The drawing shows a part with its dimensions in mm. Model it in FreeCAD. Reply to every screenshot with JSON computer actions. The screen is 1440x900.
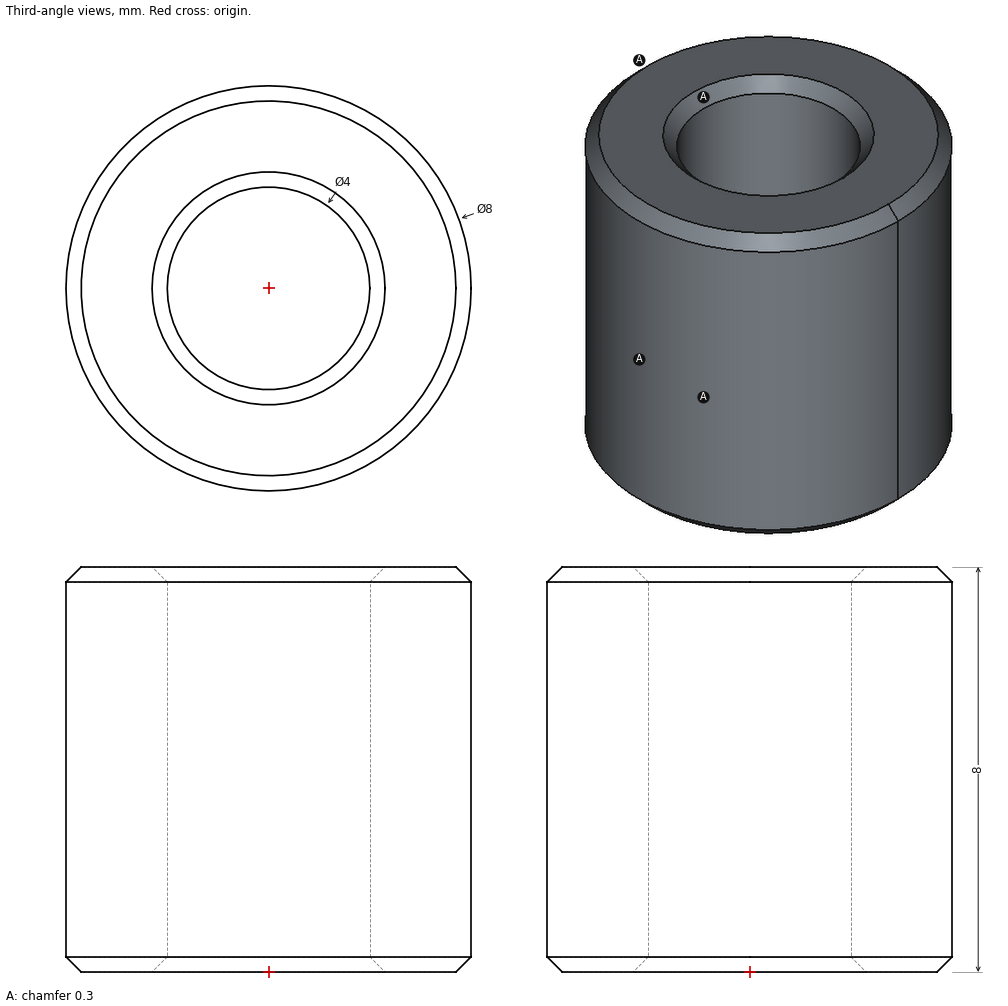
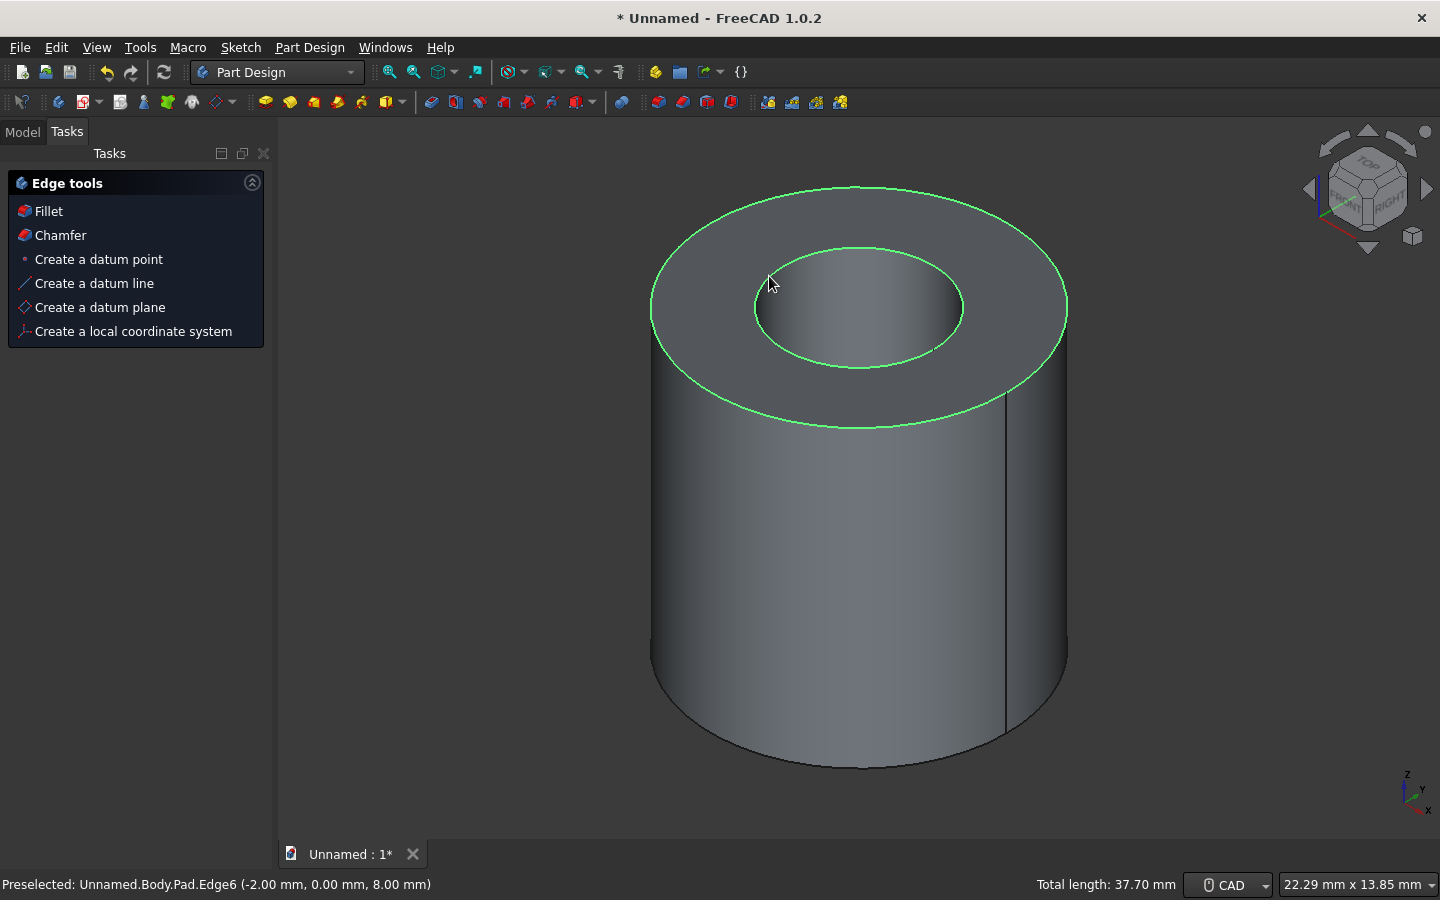
{"action": "key", "text": "2"}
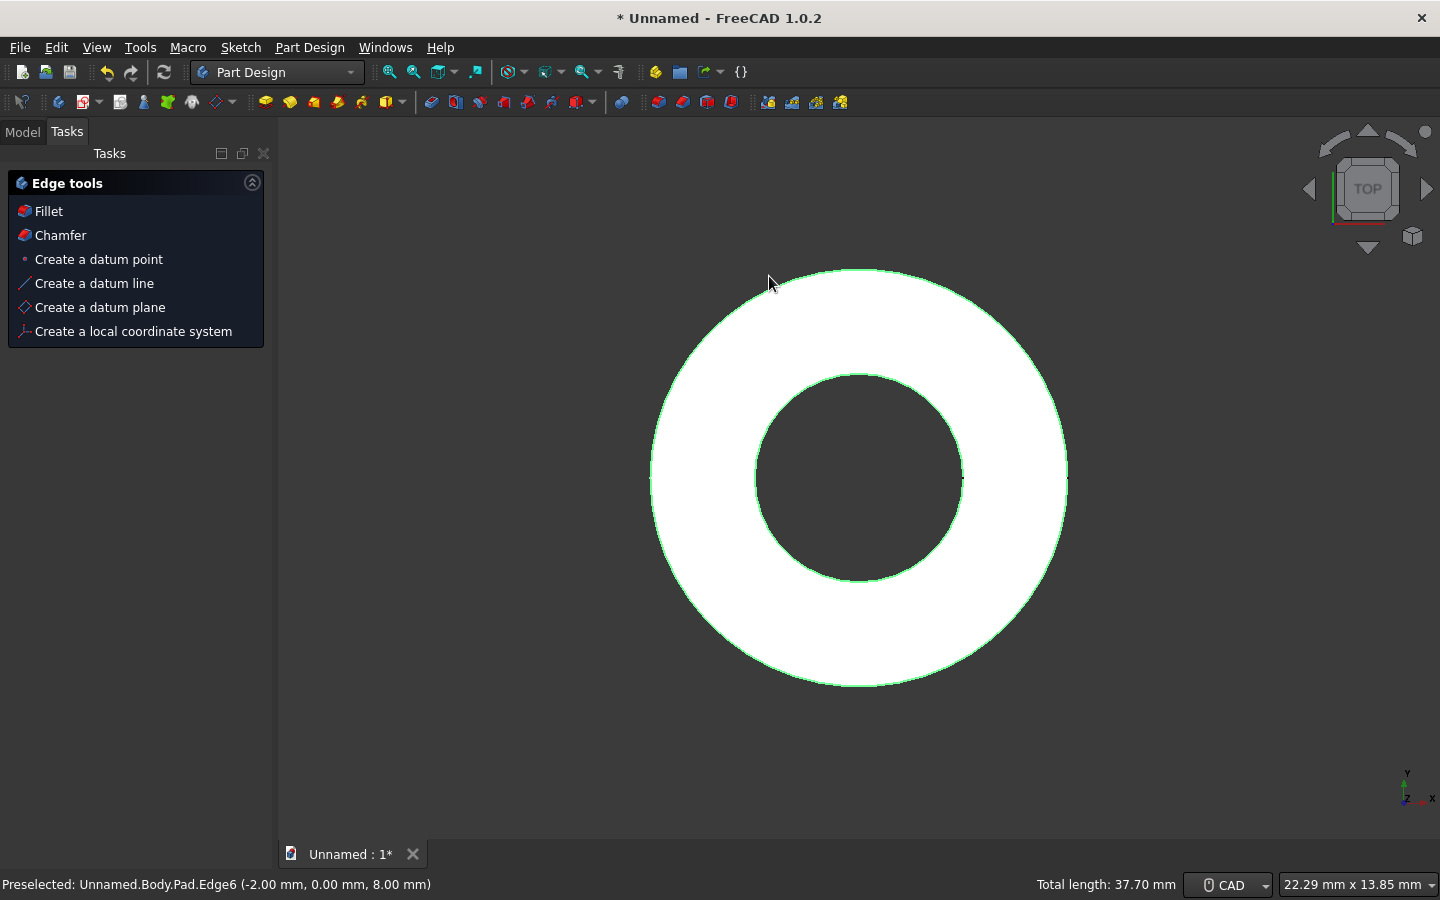
{"action": "key", "text": "1"}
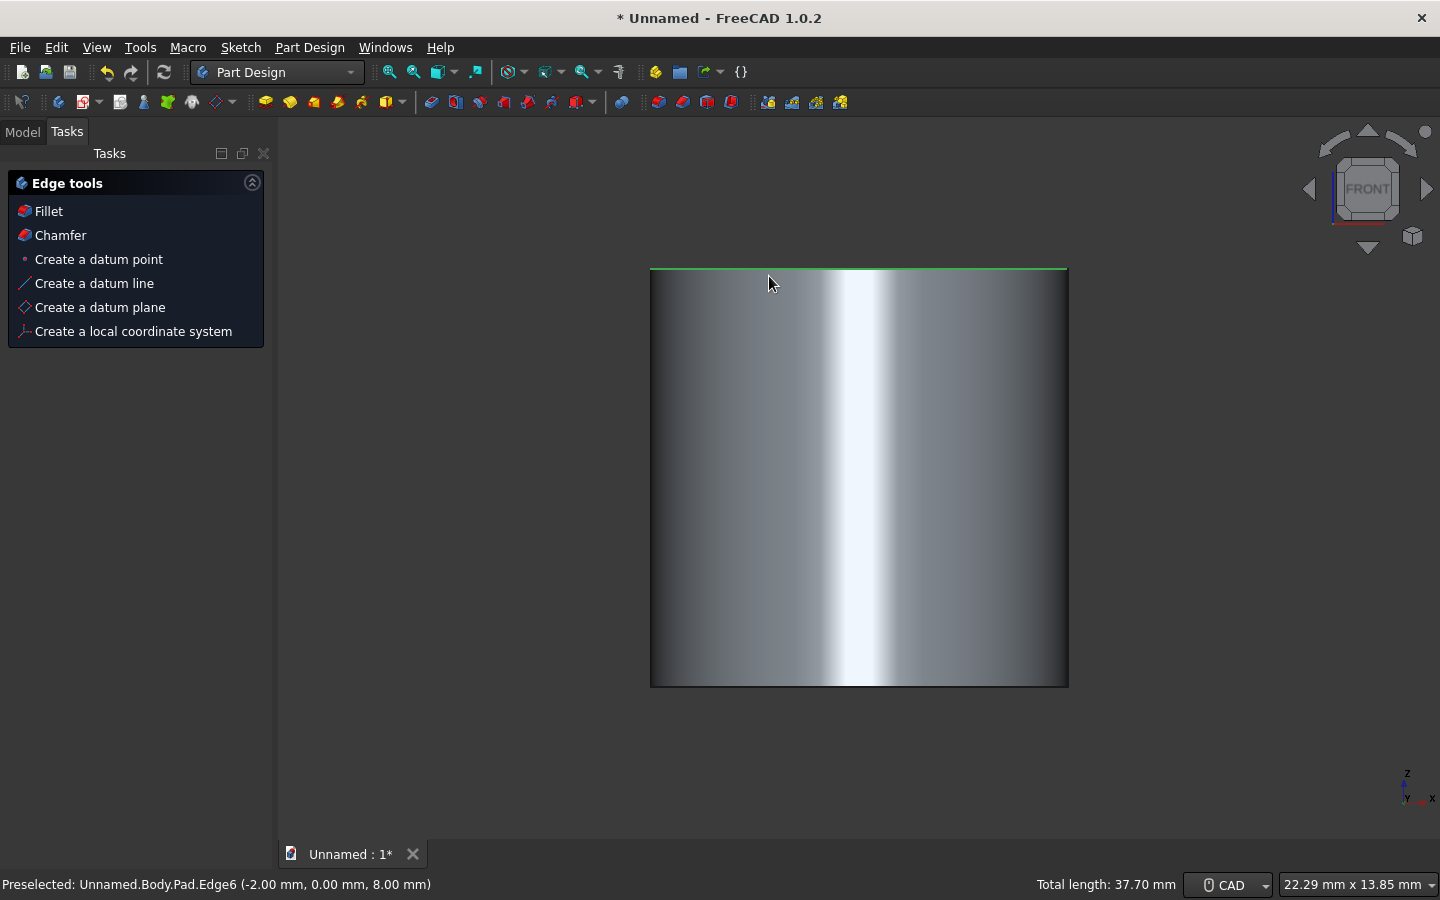
{"action": "left_click", "coordinate": [690, 686], "text": "ctrl"}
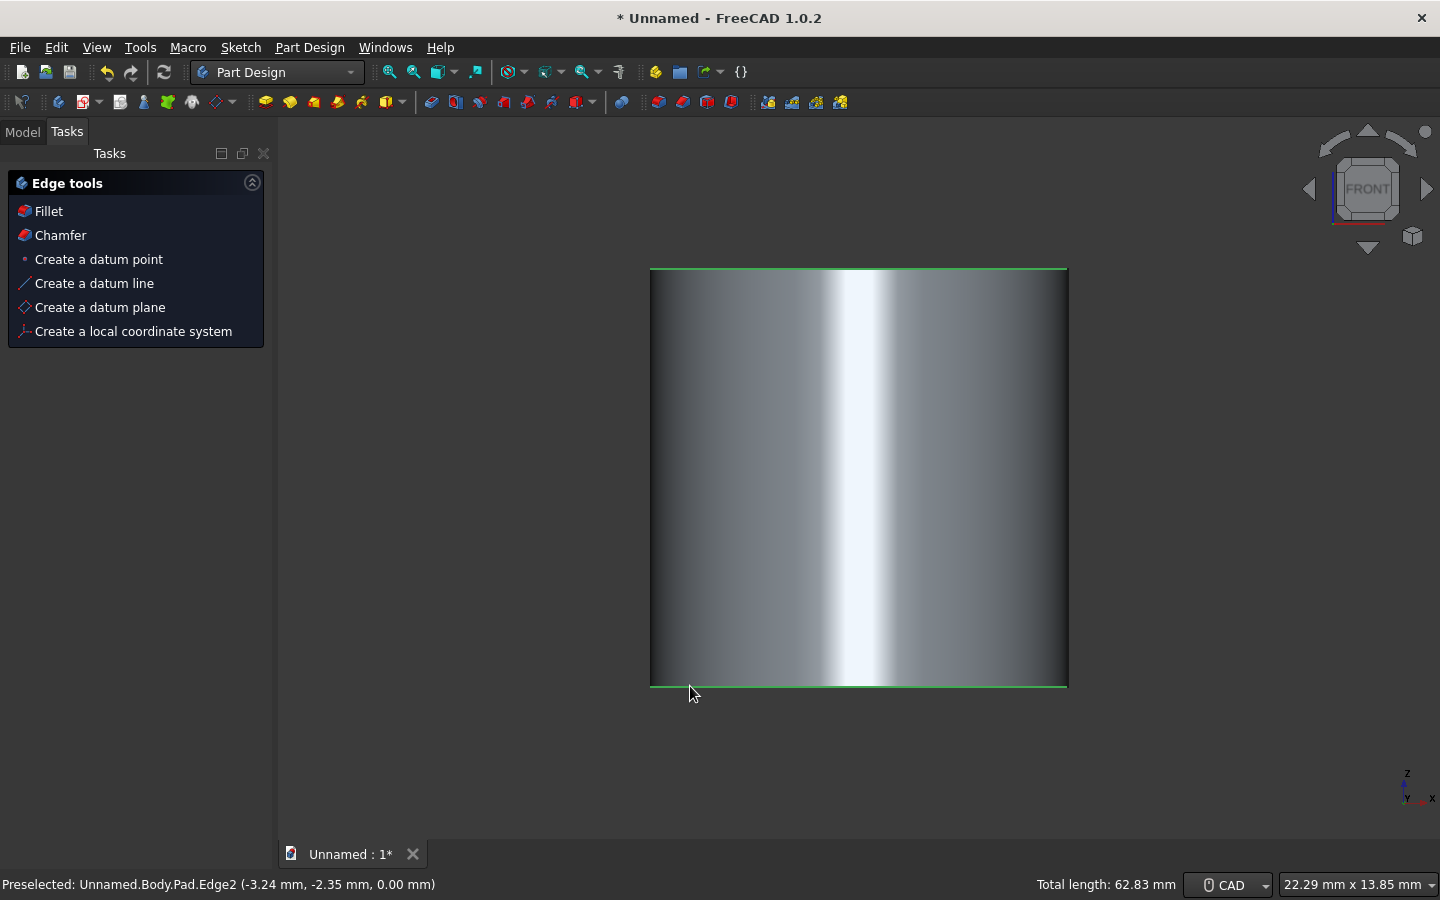
{"action": "key", "text": "3"}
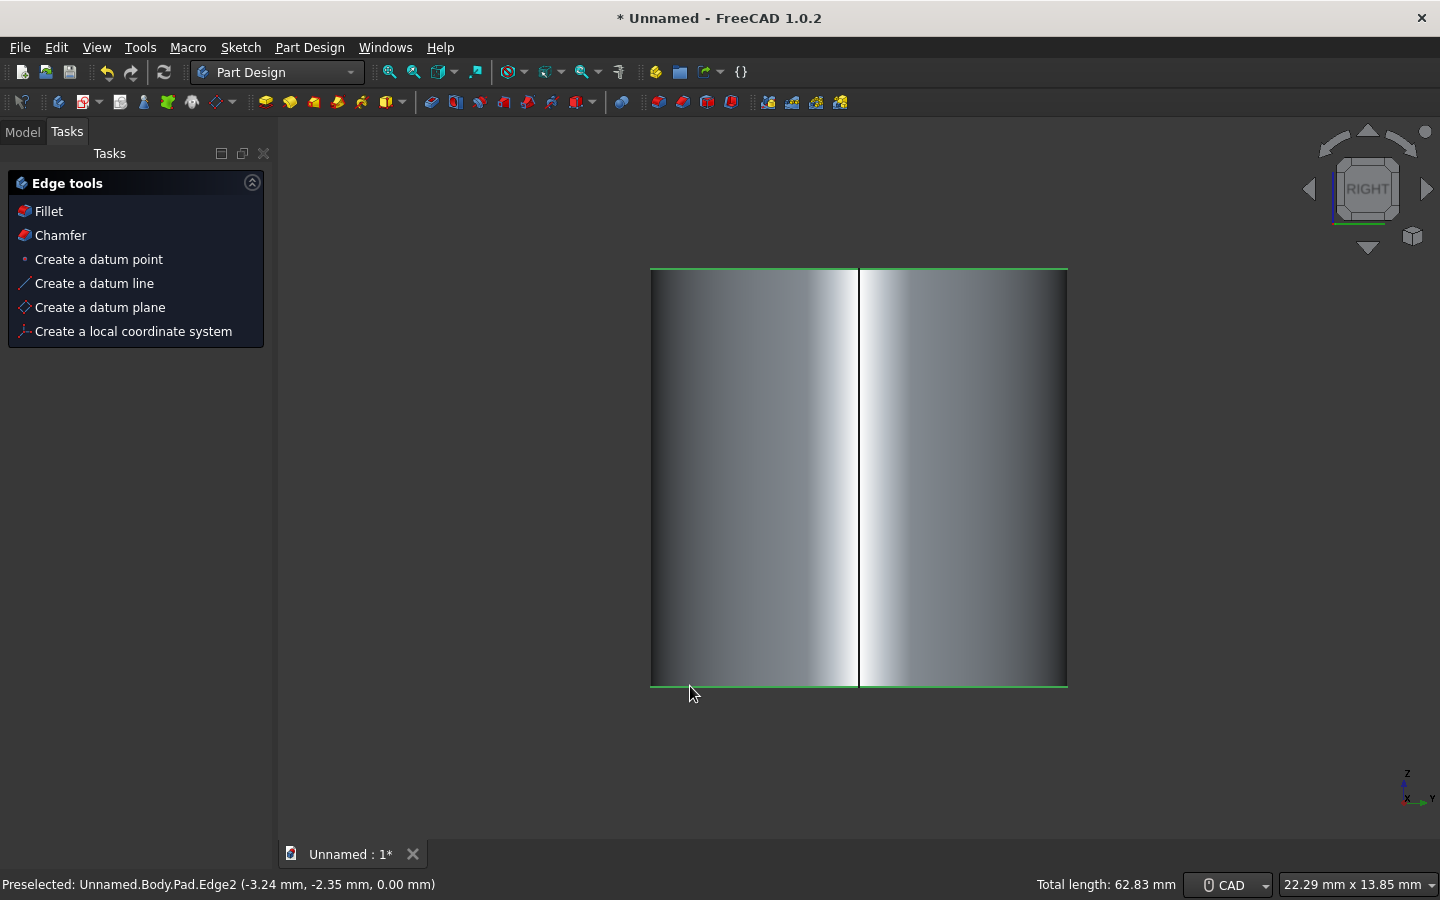
{"action": "key", "text": "5"}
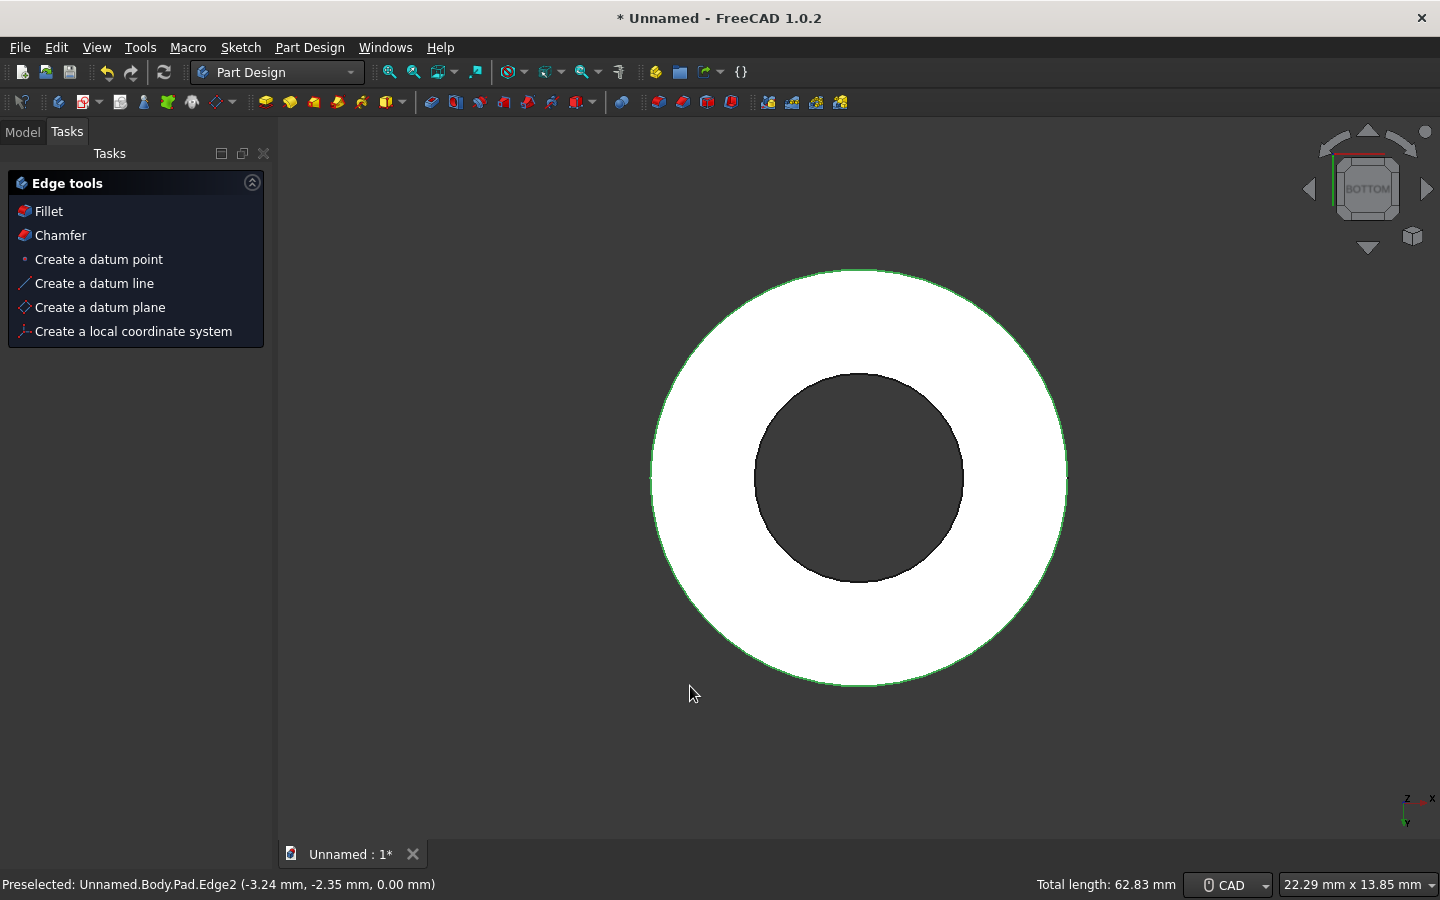
{"action": "left_click", "coordinate": [755, 477], "text": "ctrl"}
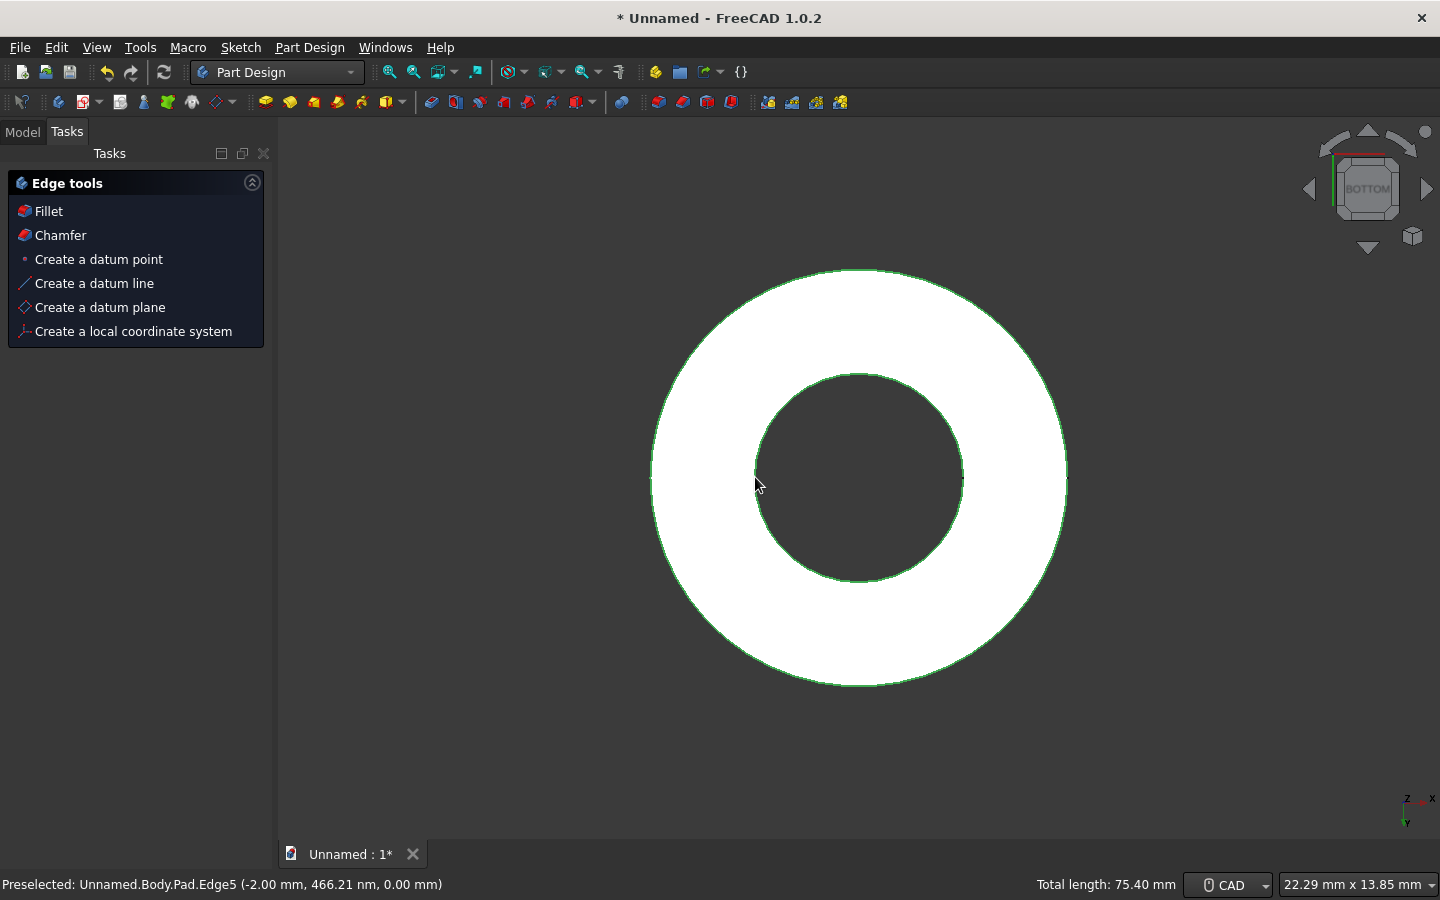
{"action": "left_click", "coordinate": [684, 102]}